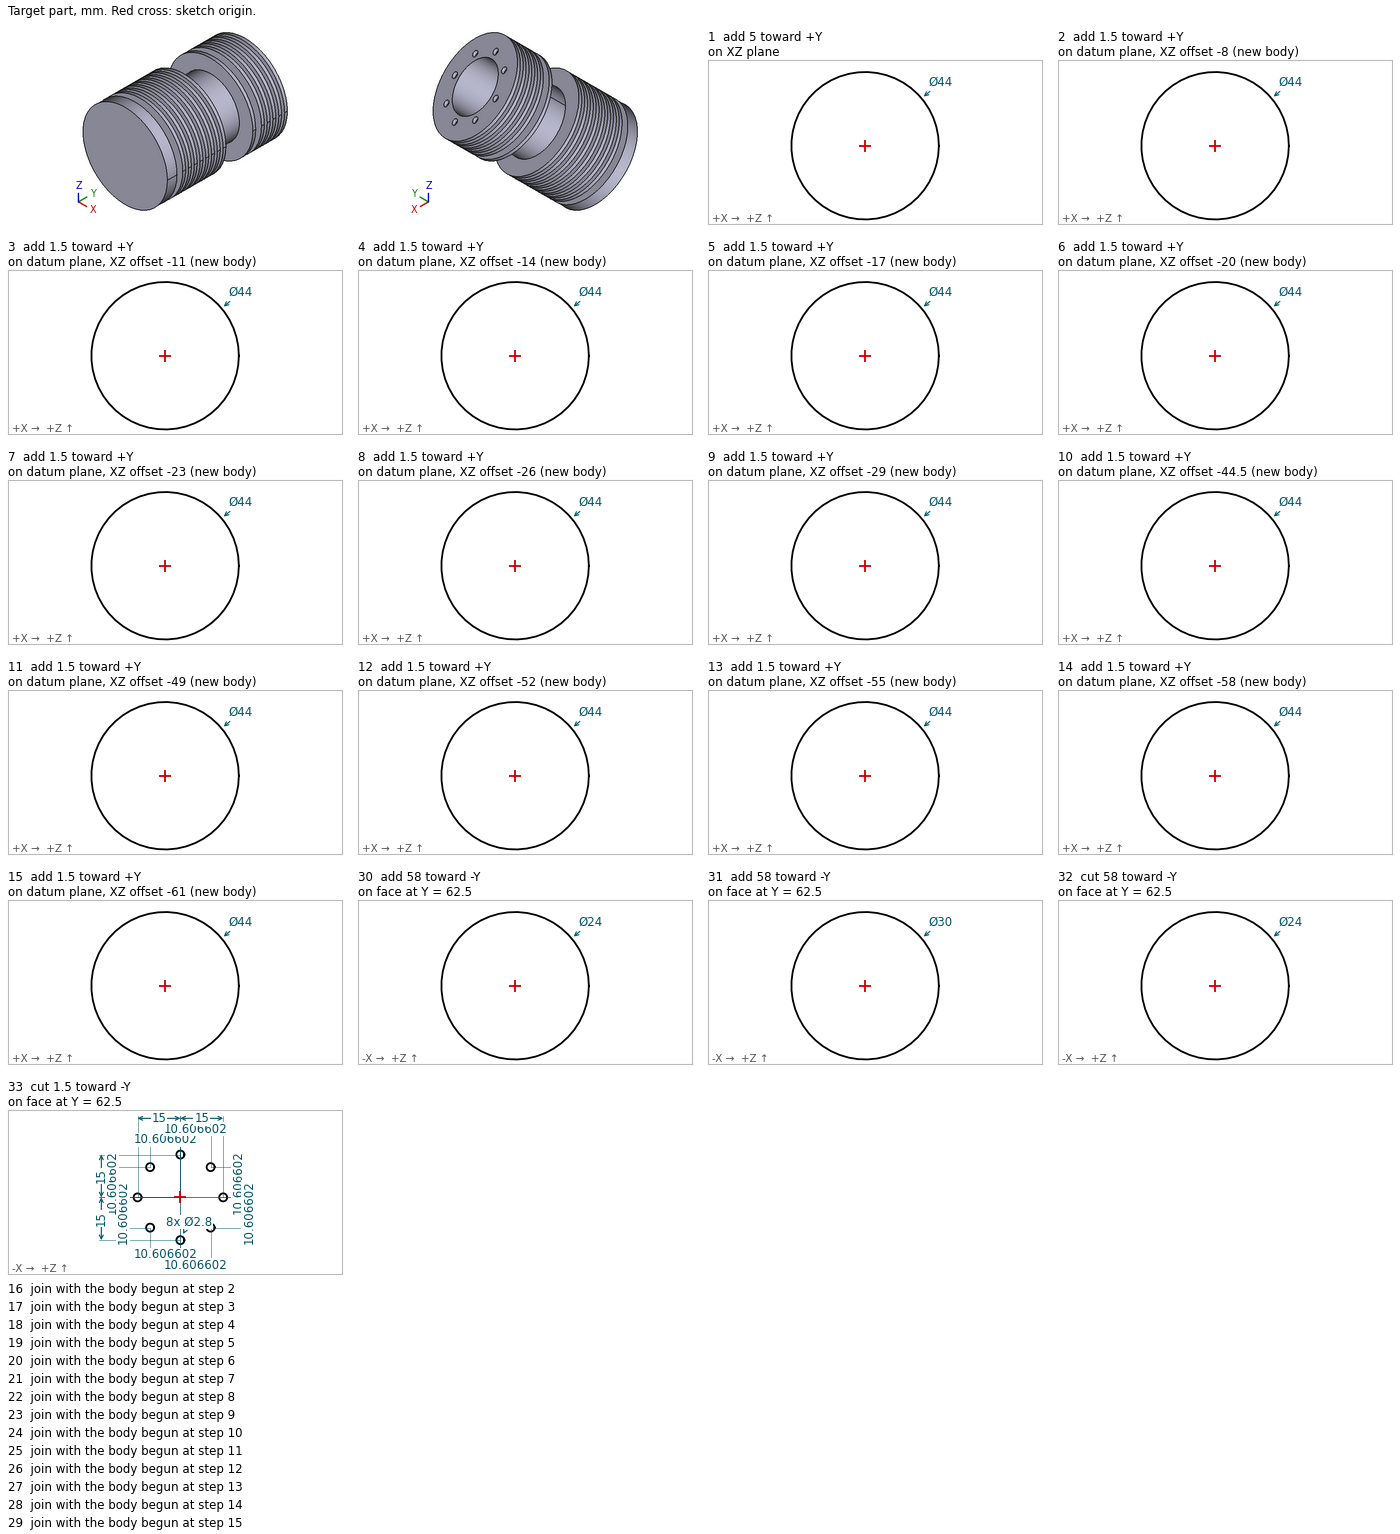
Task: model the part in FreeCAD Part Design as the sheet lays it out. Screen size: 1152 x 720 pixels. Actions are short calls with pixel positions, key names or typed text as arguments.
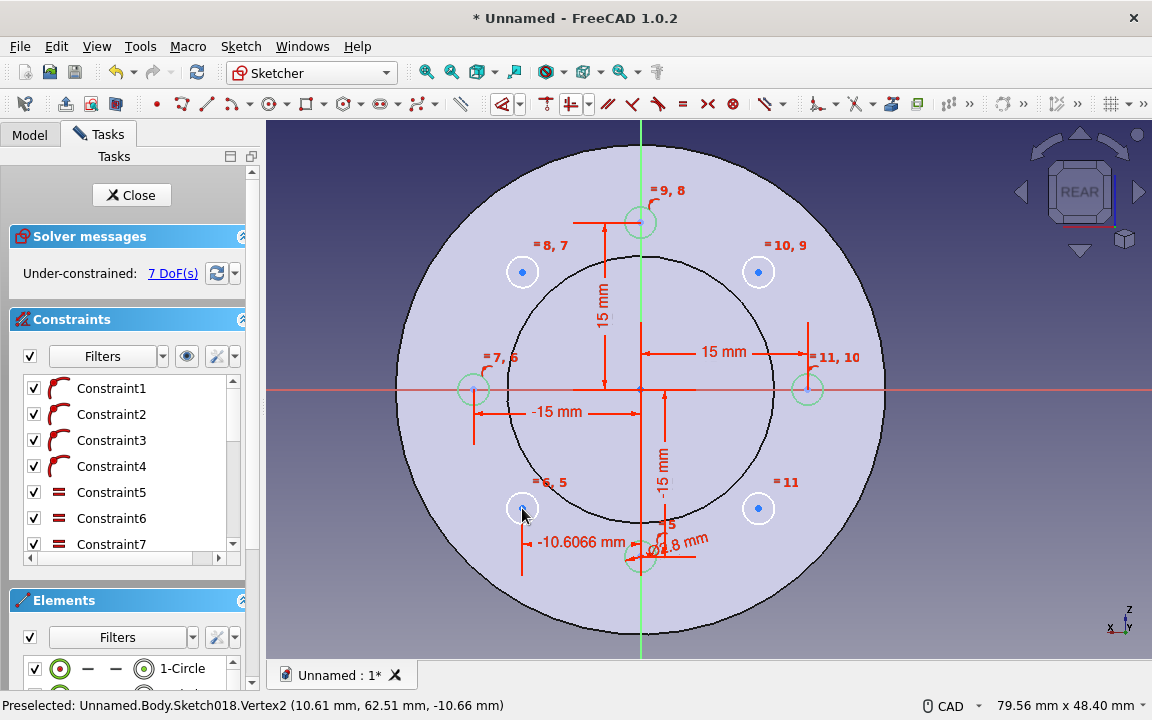
click(522, 508)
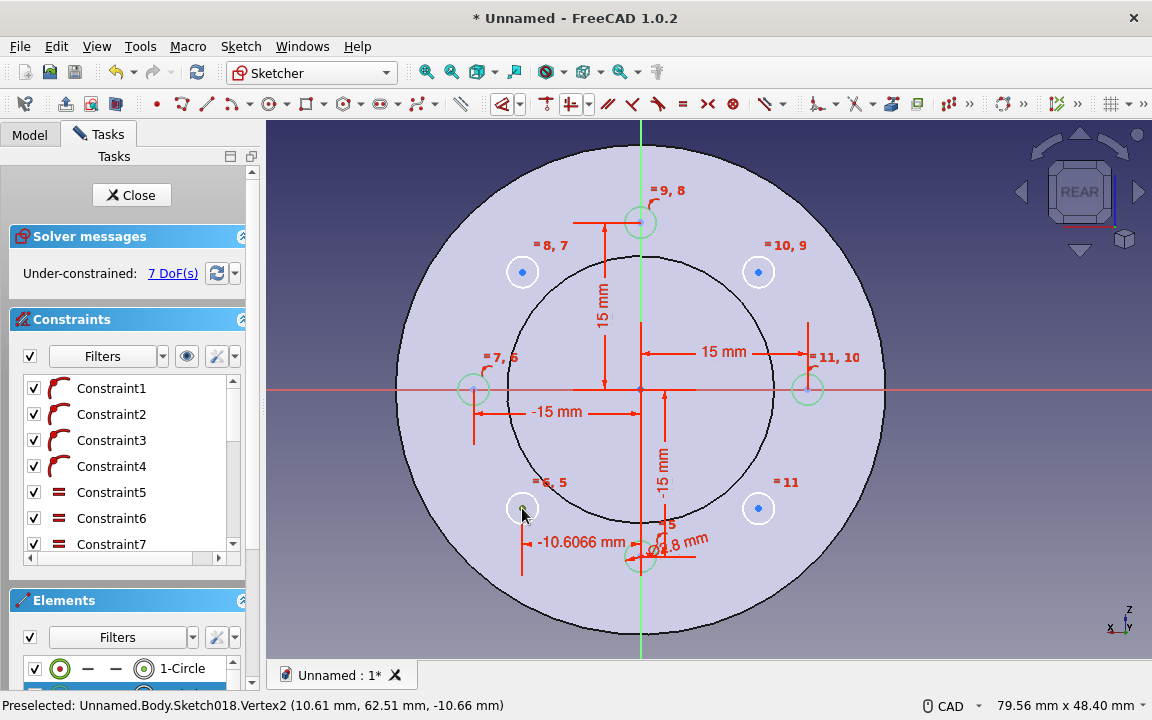
key(i)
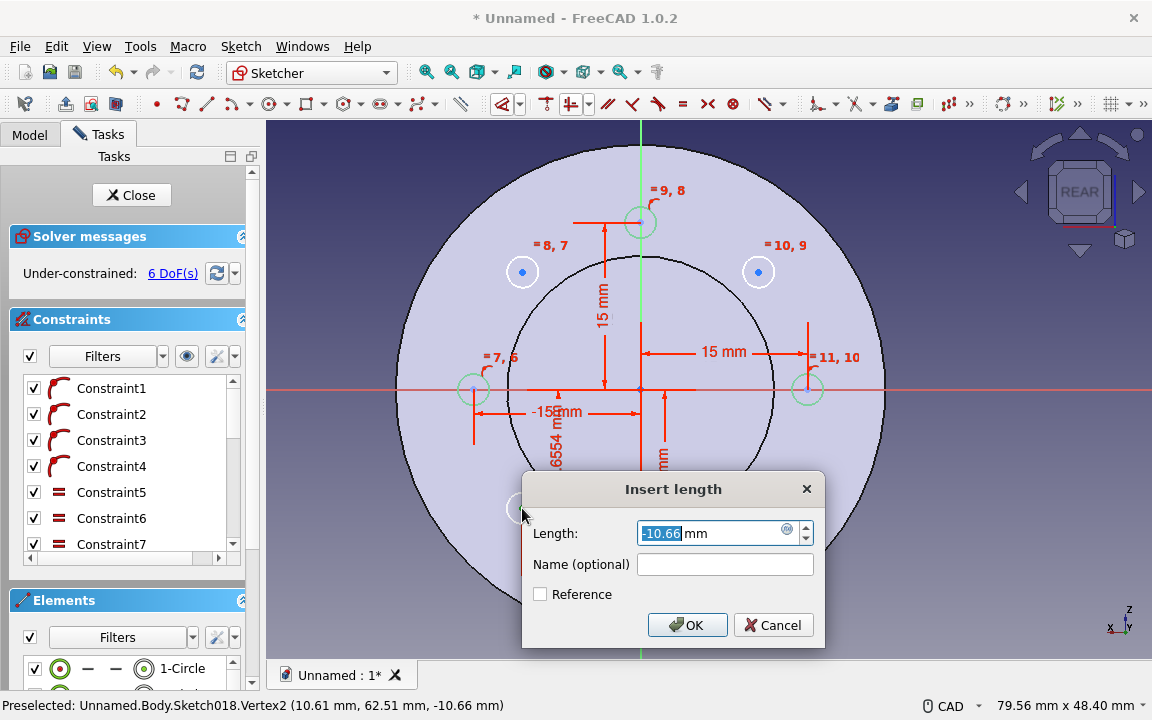
text(-10.606602)
key(Return)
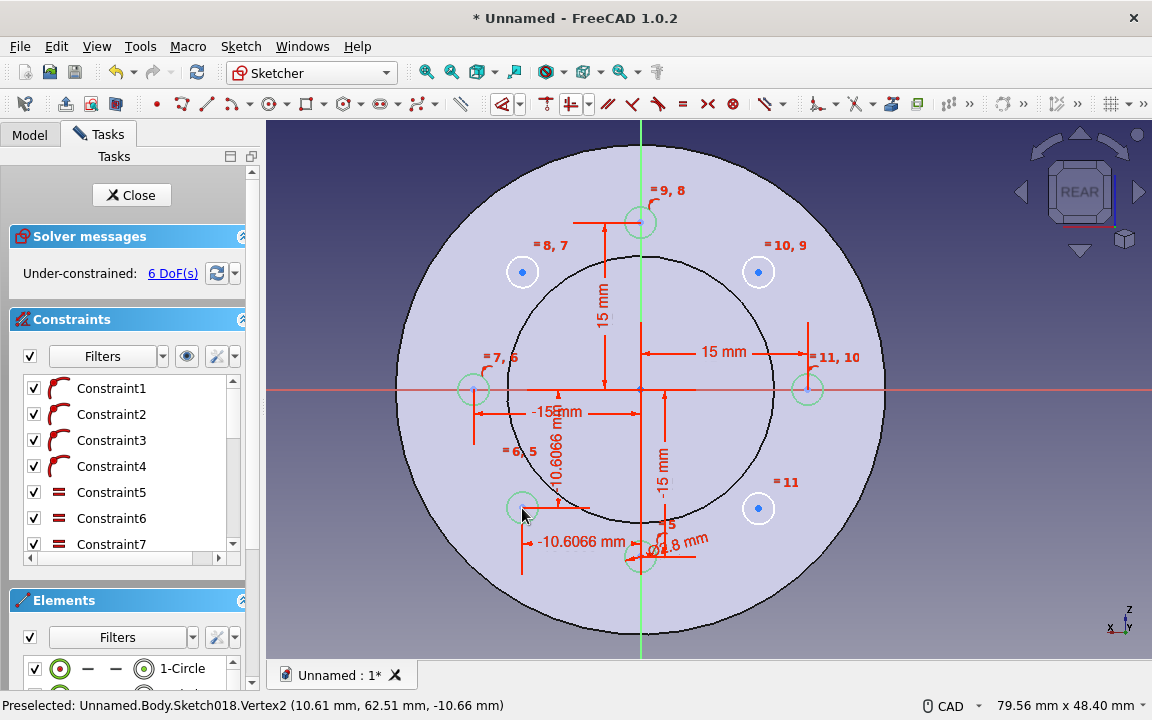
click(523, 272)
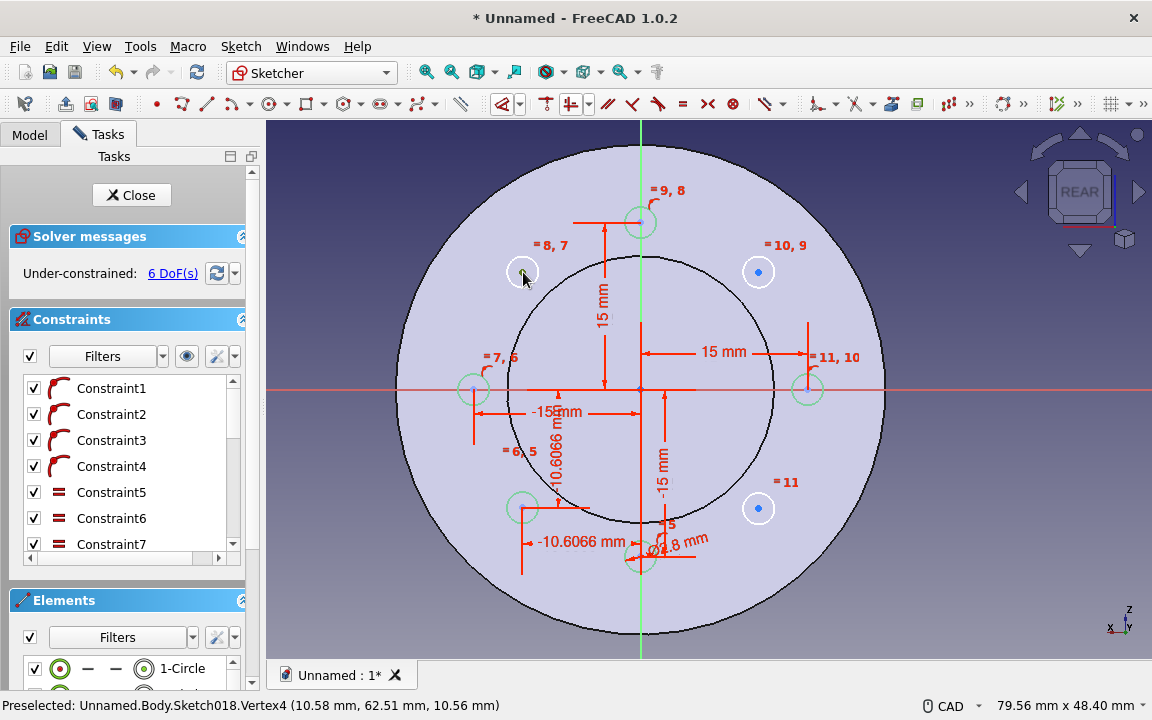
key(l)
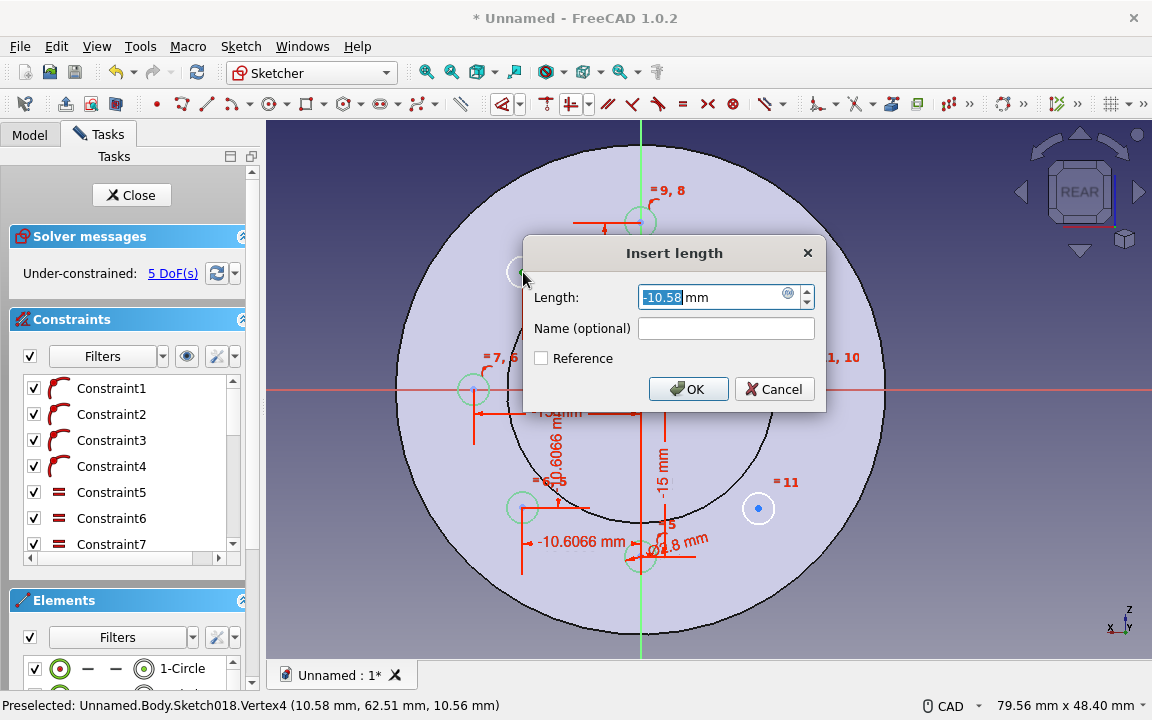
text(-10.606602)
key(Return)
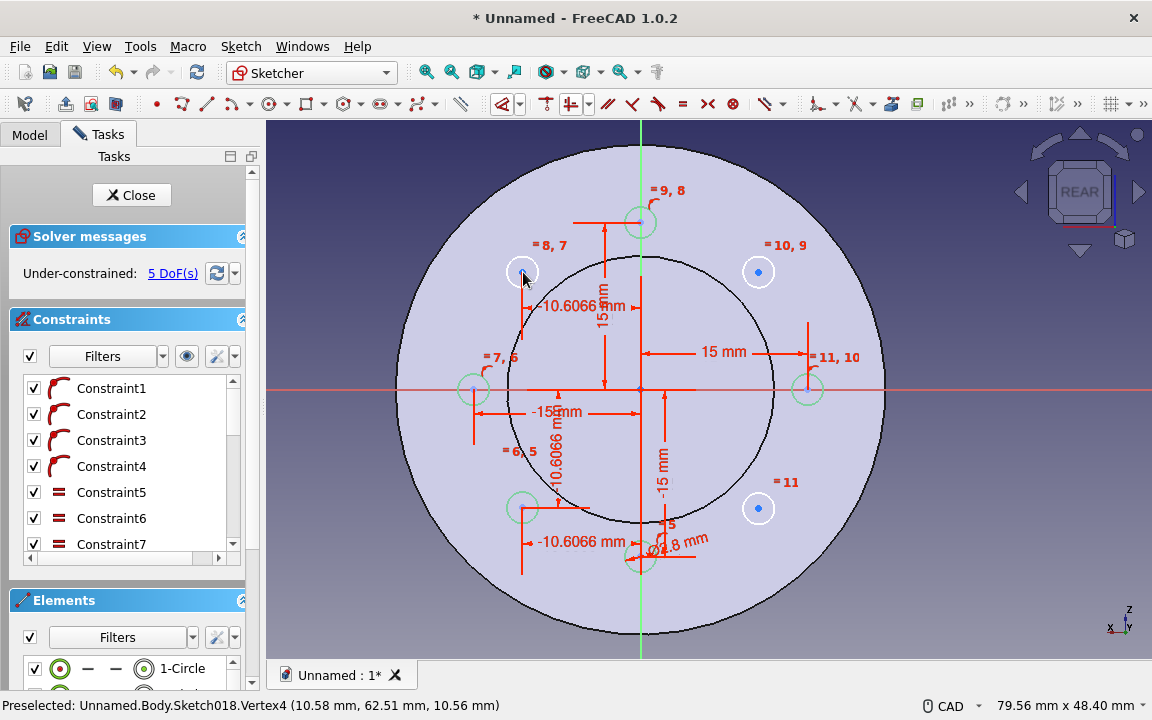
click(522, 272)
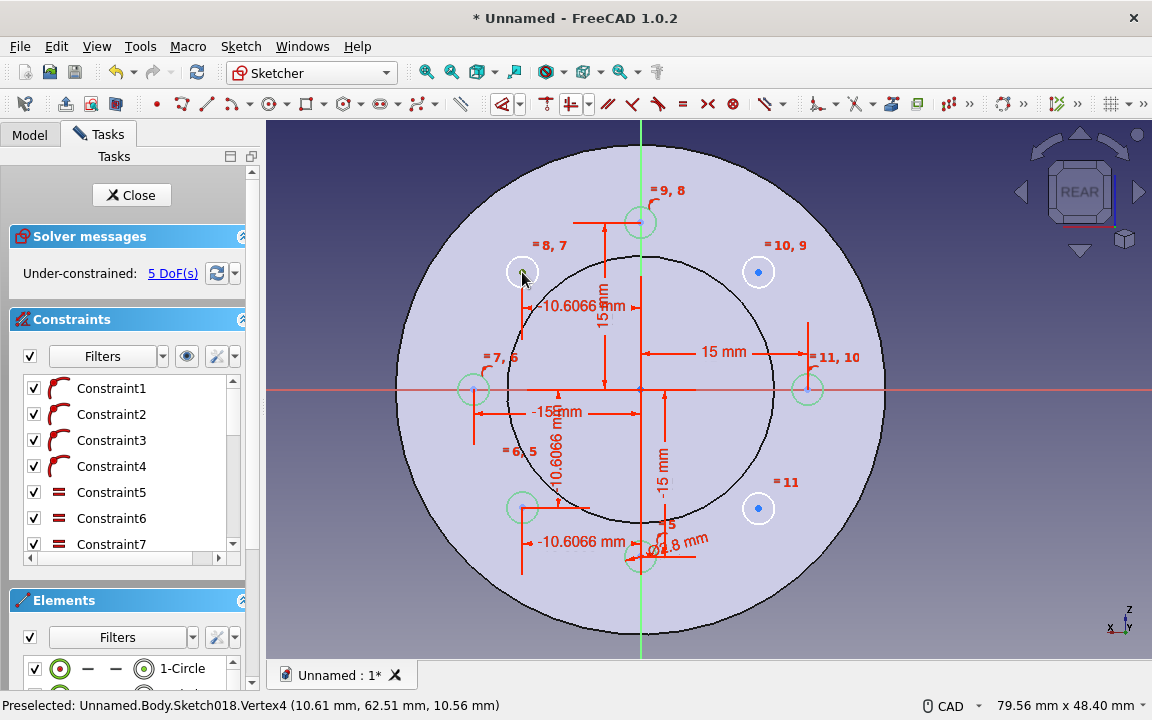
key(i)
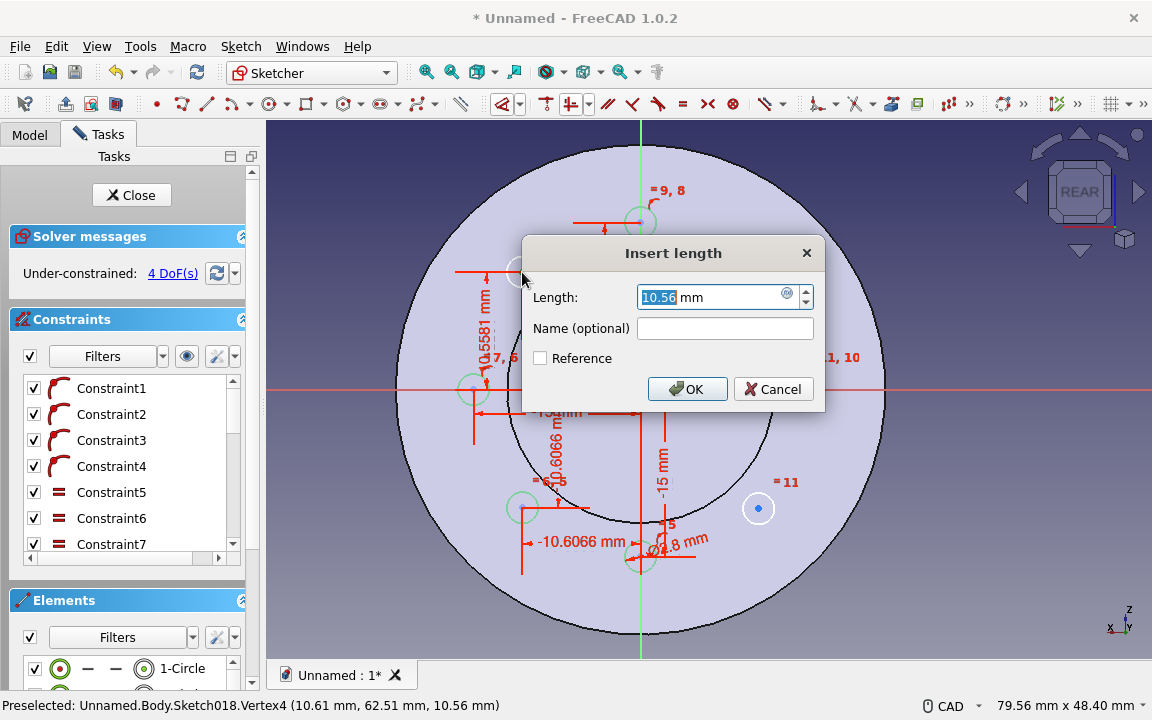
text(10.606602)
key(Return)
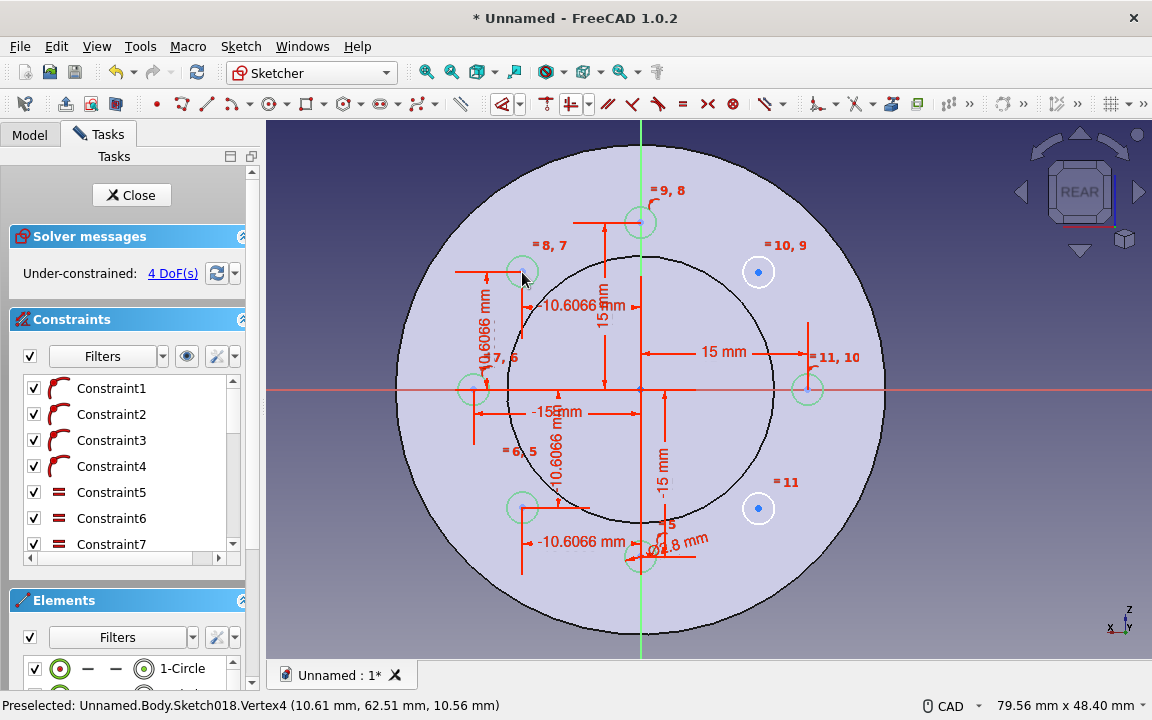
click(759, 272)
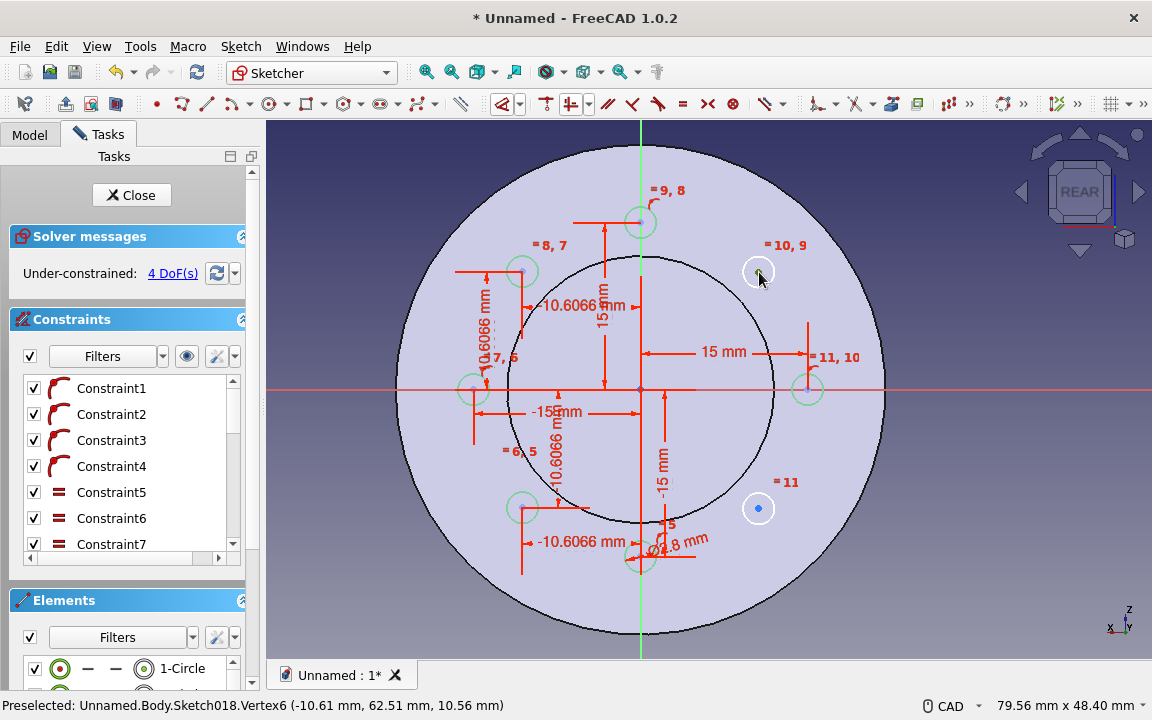
click(520, 104)